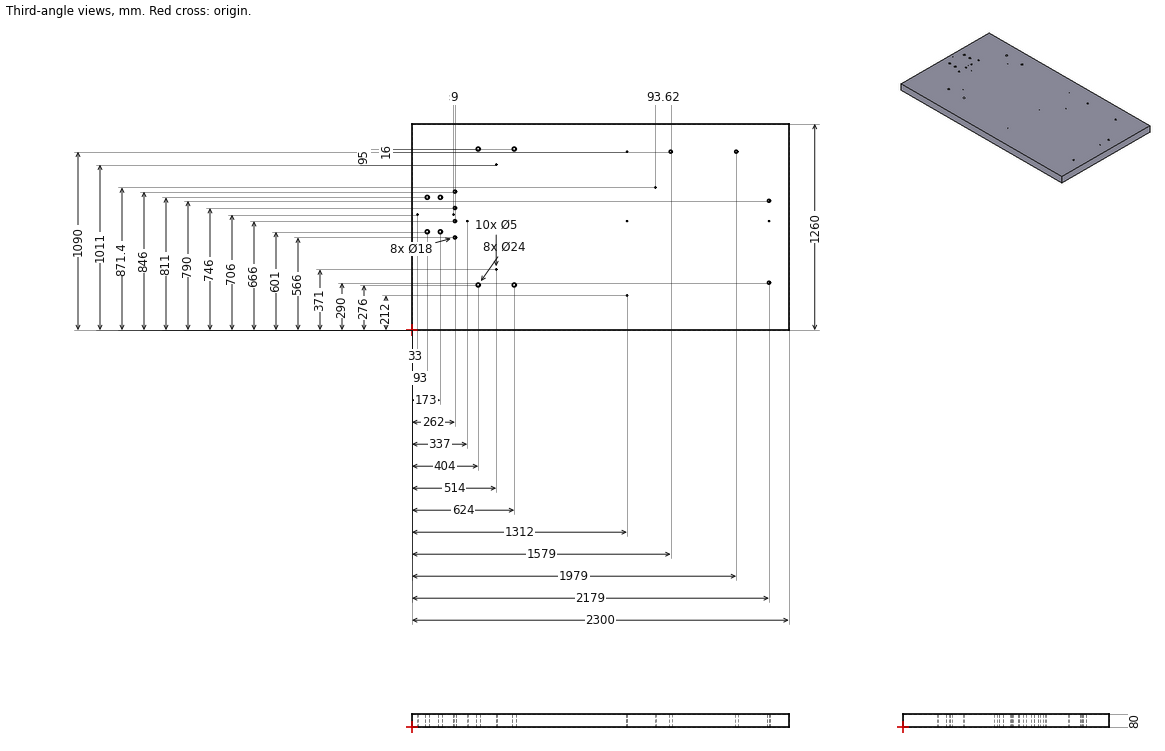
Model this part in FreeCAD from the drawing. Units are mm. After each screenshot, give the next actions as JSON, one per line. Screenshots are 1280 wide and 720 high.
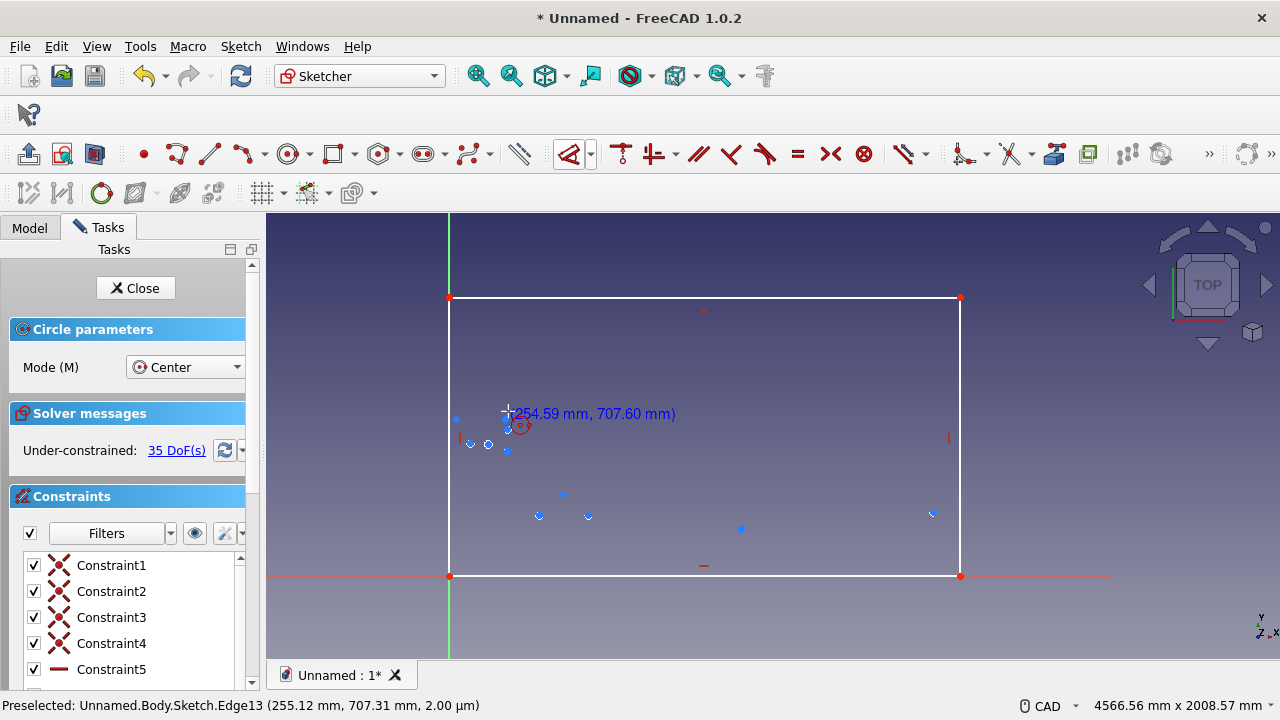
{"action": "scroll", "coordinate": [508, 411], "scroll_direction": "up", "scroll_amount": 4}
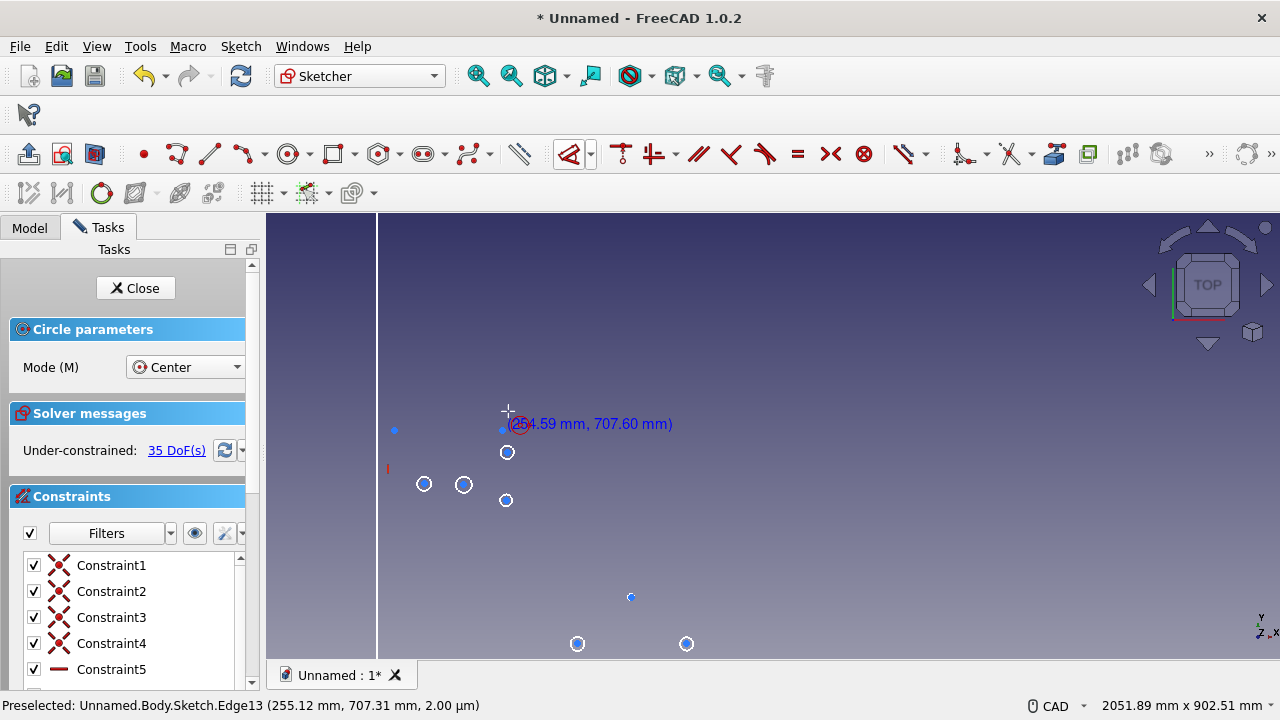
{"action": "left_click", "coordinate": [507, 410]}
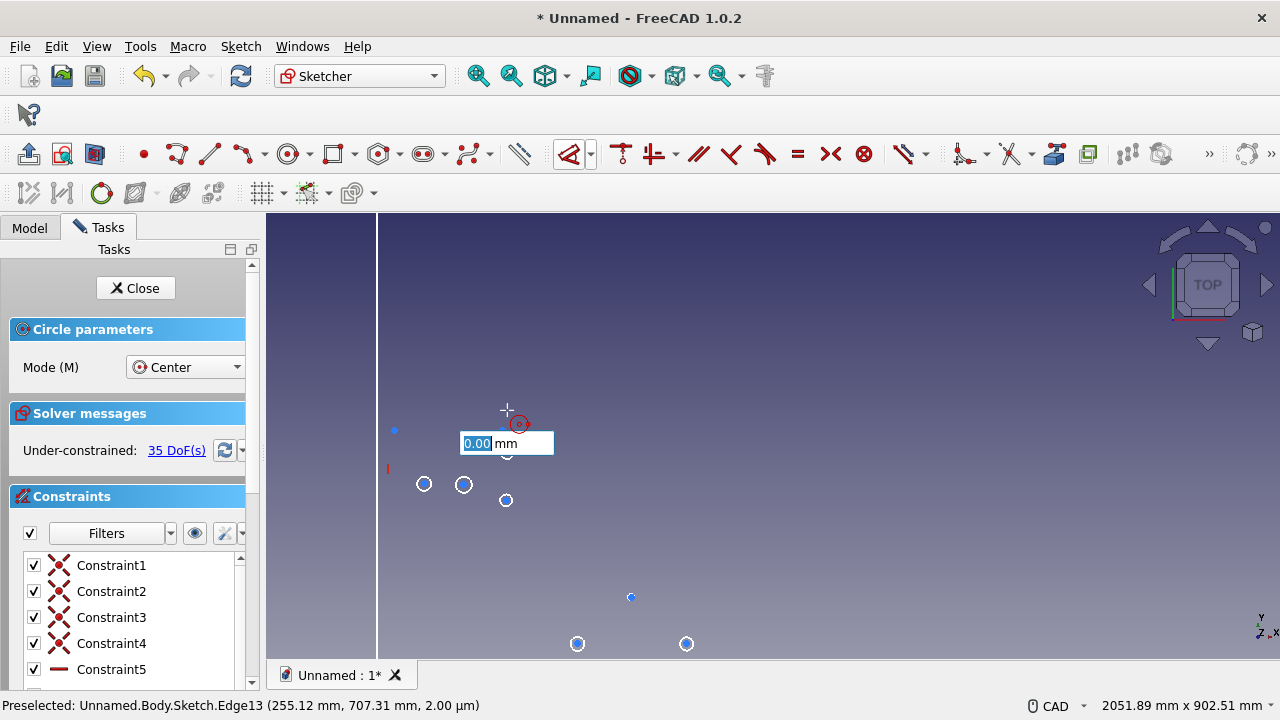
{"action": "scroll", "coordinate": [510, 407], "scroll_direction": "up", "scroll_amount": 7}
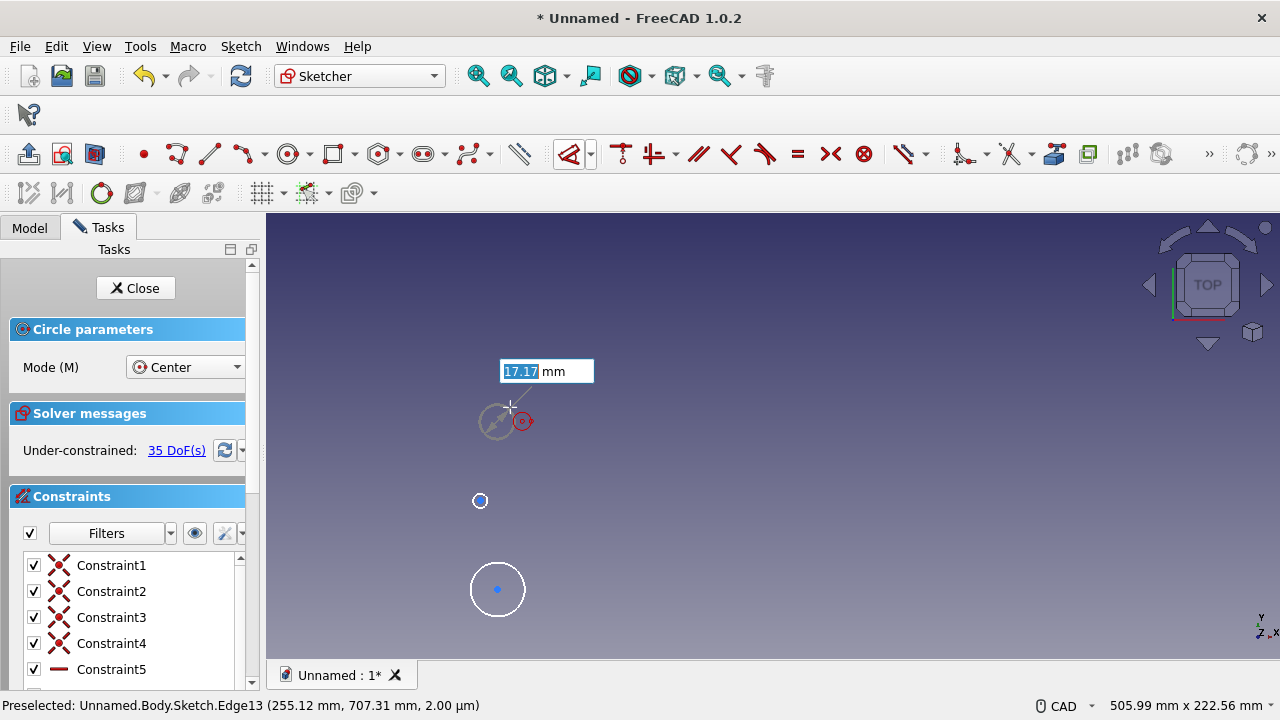
{"action": "left_click", "coordinate": [510, 404]}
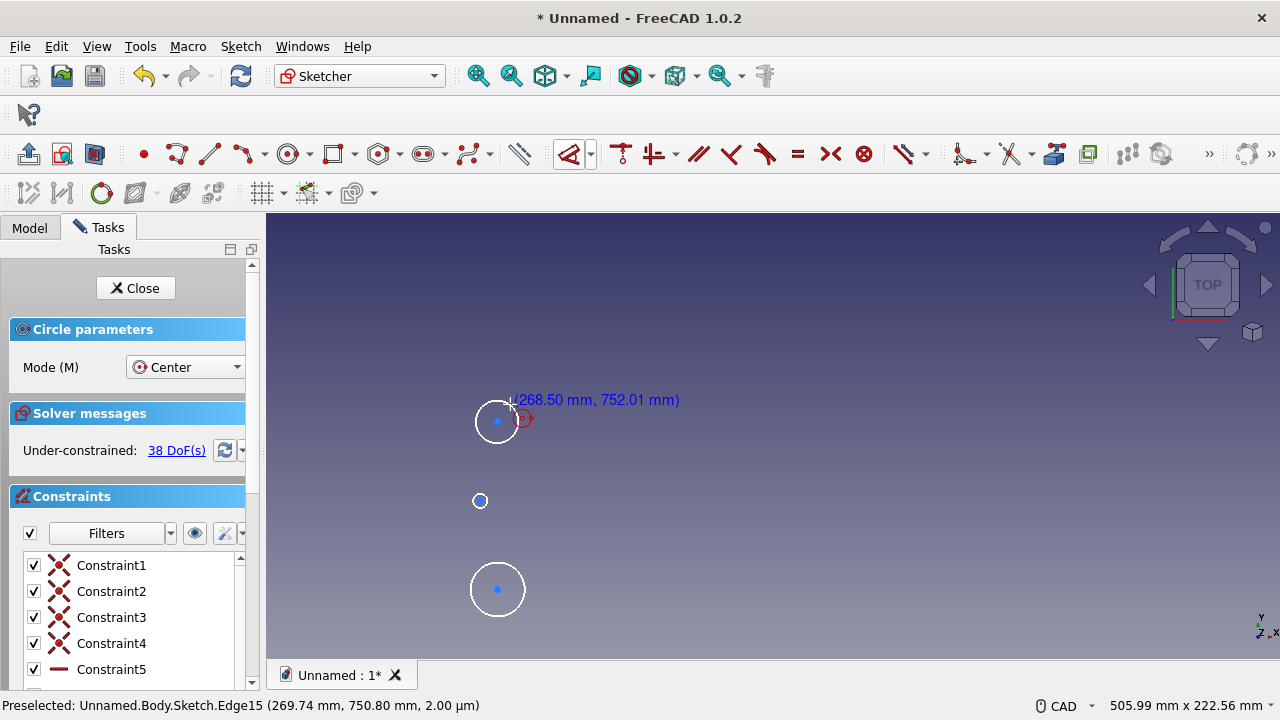
{"action": "scroll", "coordinate": [647, 577], "scroll_direction": "up", "scroll_amount": 8}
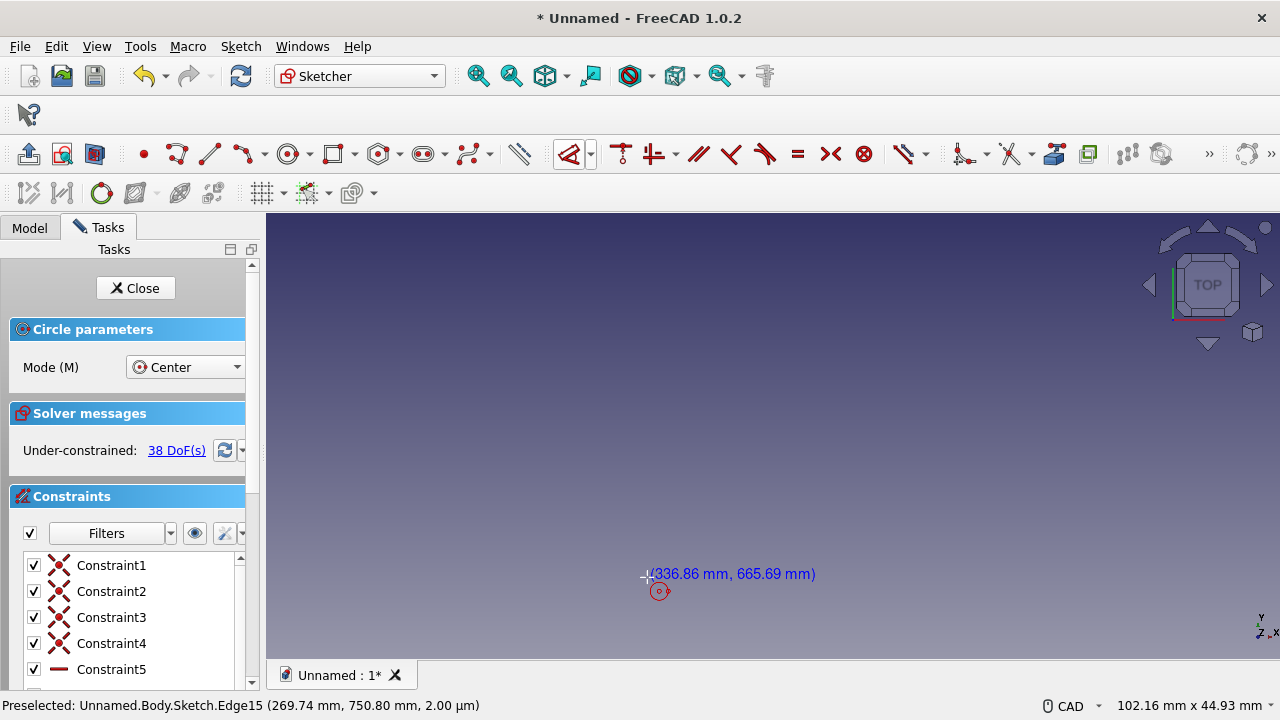
{"action": "scroll", "coordinate": [704, 436], "scroll_direction": "down", "scroll_amount": 15}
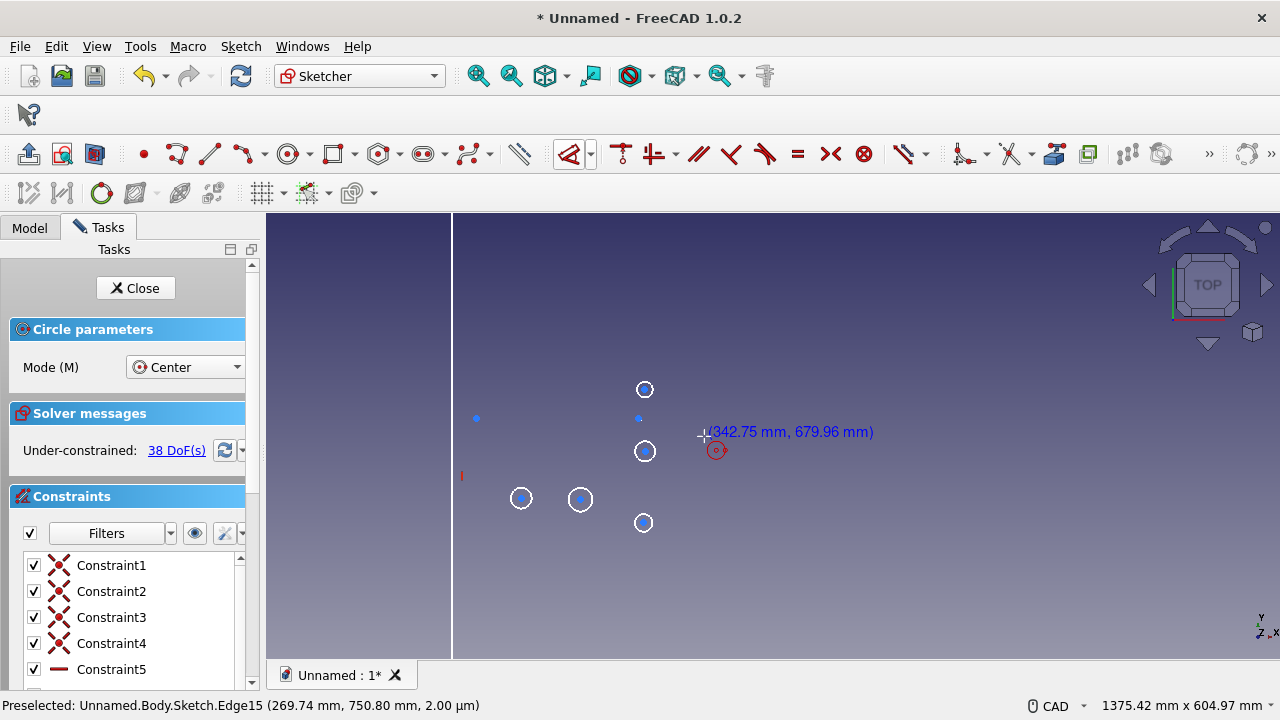
{"action": "scroll", "coordinate": [379, 415], "scroll_direction": "down", "scroll_amount": 4}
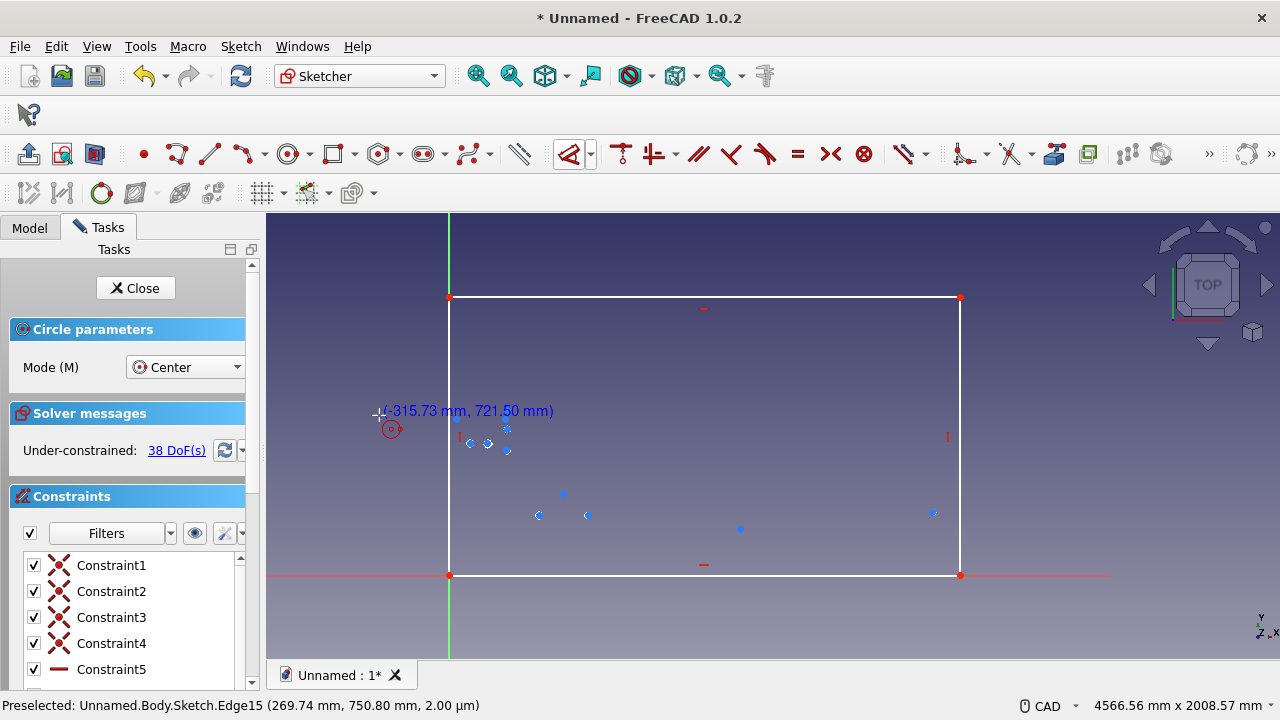
{"action": "left_click", "coordinate": [524, 428]}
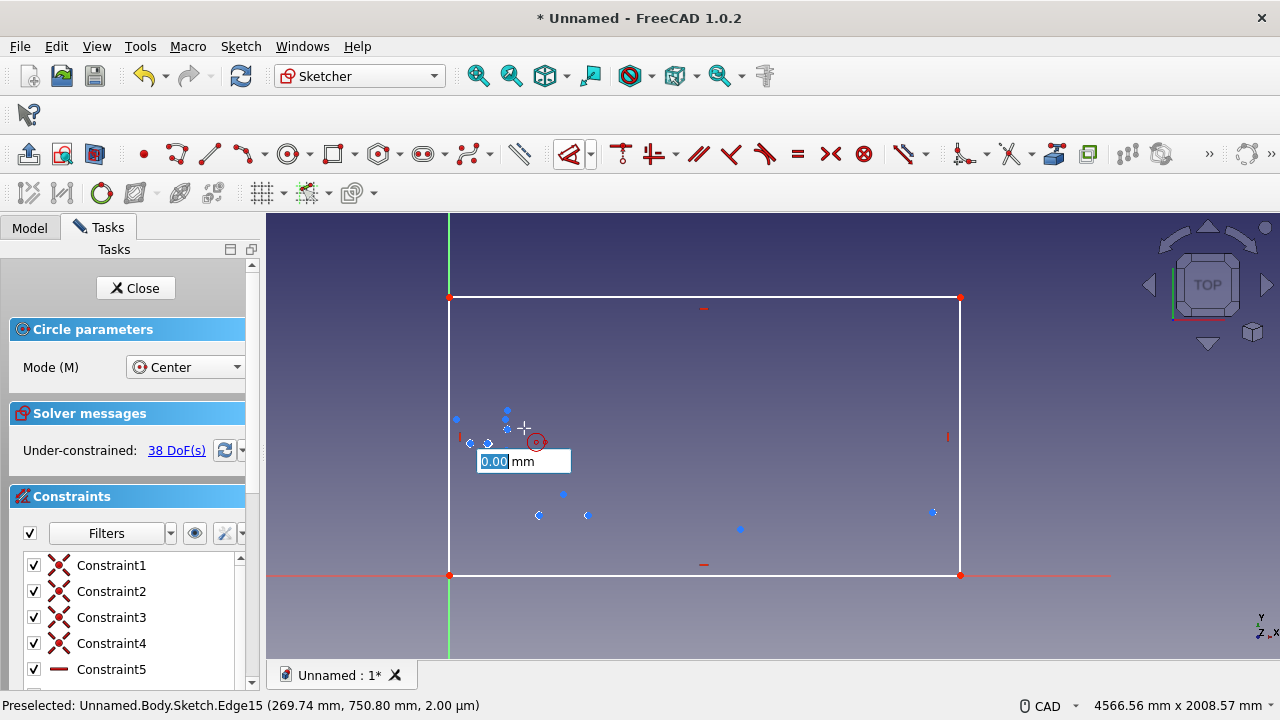
{"action": "scroll", "coordinate": [524, 428], "scroll_direction": "up", "scroll_amount": 17}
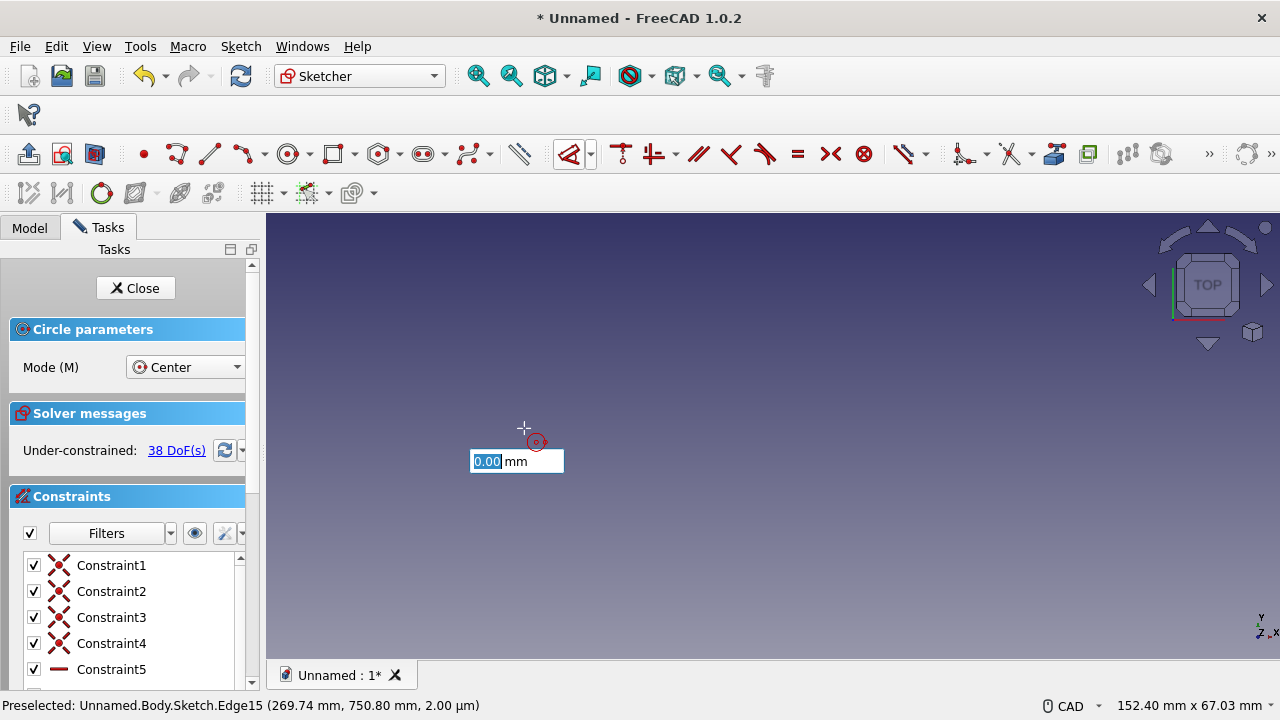
{"action": "left_click", "coordinate": [528, 403]}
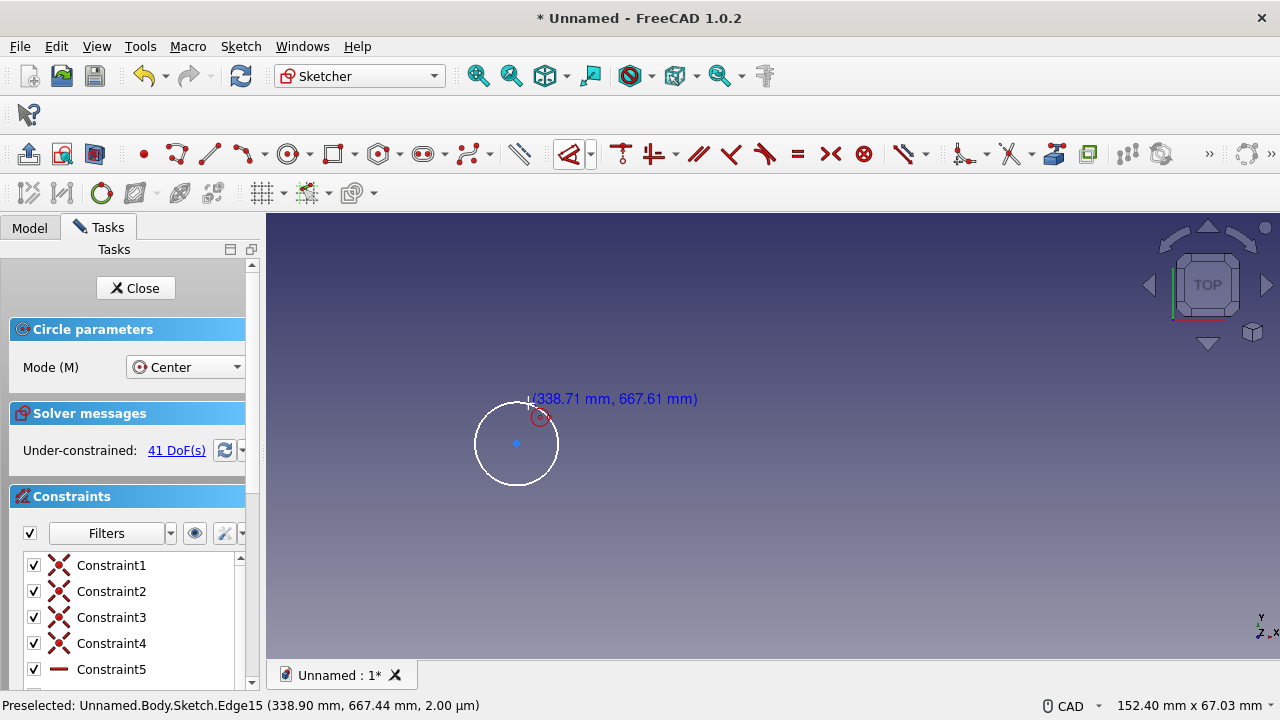
{"action": "scroll", "coordinate": [524, 428], "scroll_direction": "down", "scroll_amount": 17}